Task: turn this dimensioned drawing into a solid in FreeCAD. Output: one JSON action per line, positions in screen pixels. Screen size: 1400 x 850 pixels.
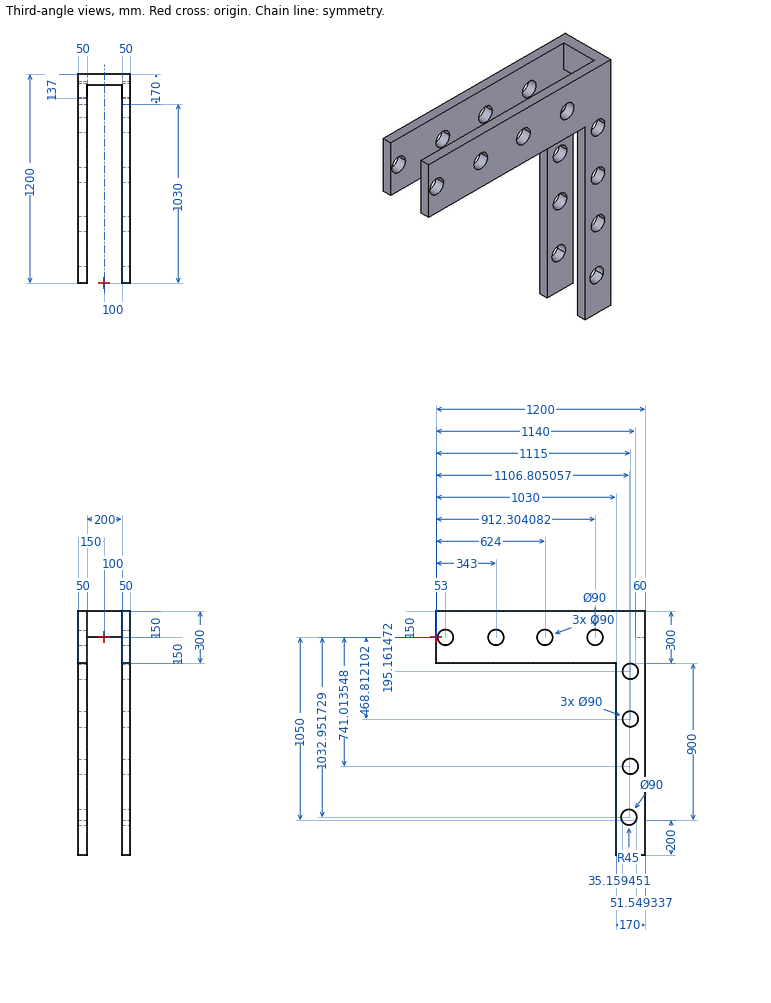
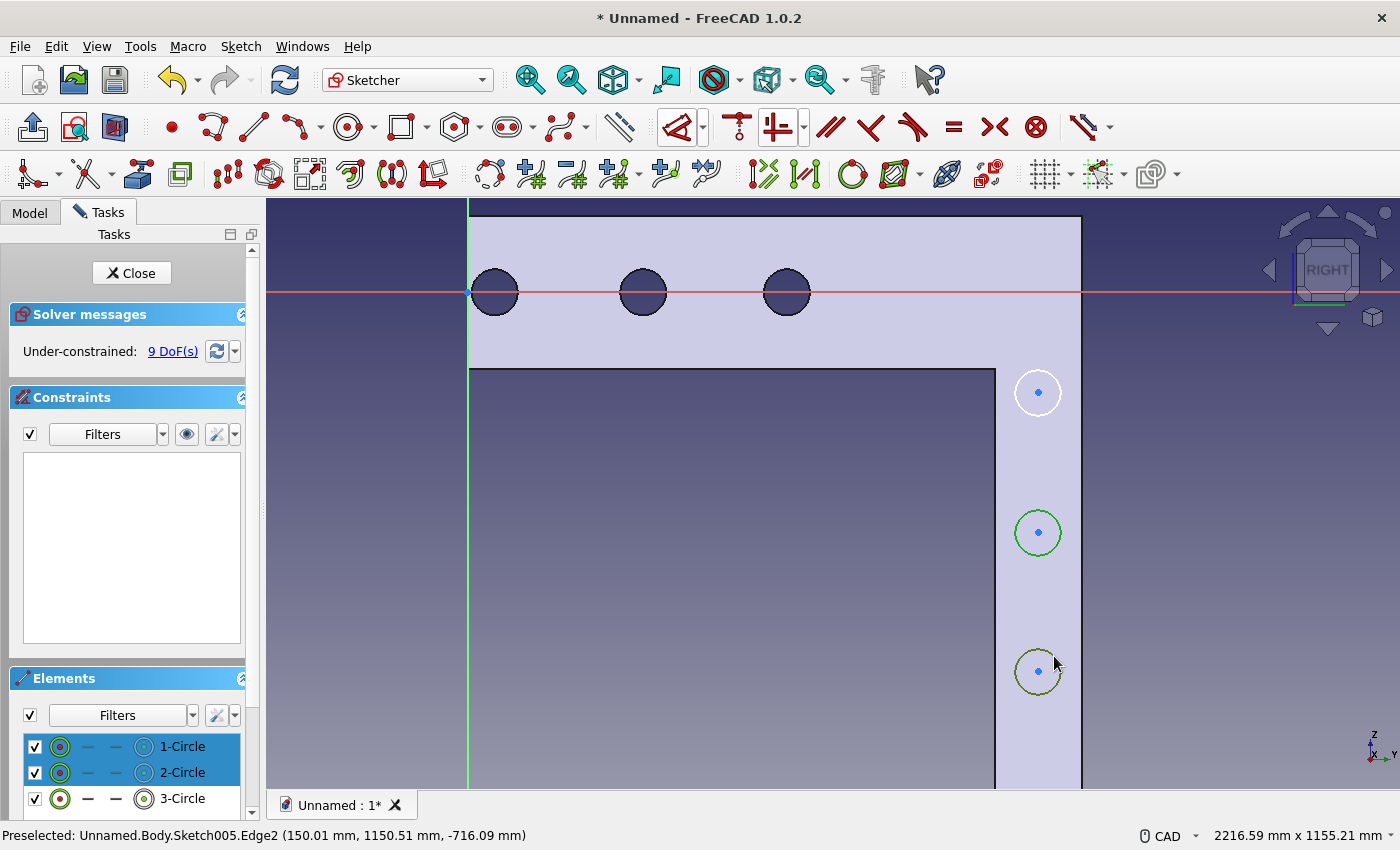
{"action": "left_click", "coordinate": [1054, 377]}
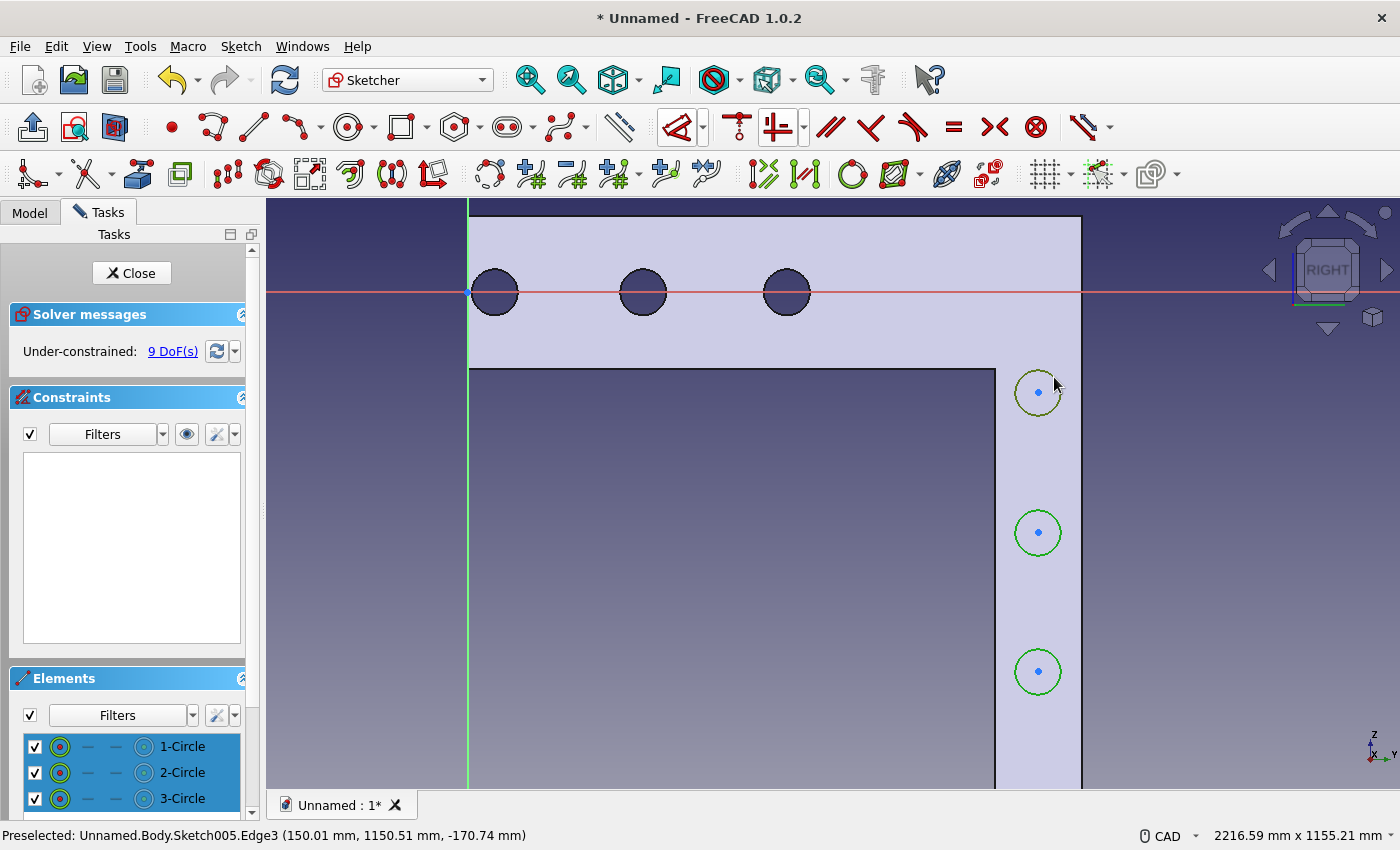
{"action": "left_click", "coordinate": [954, 128]}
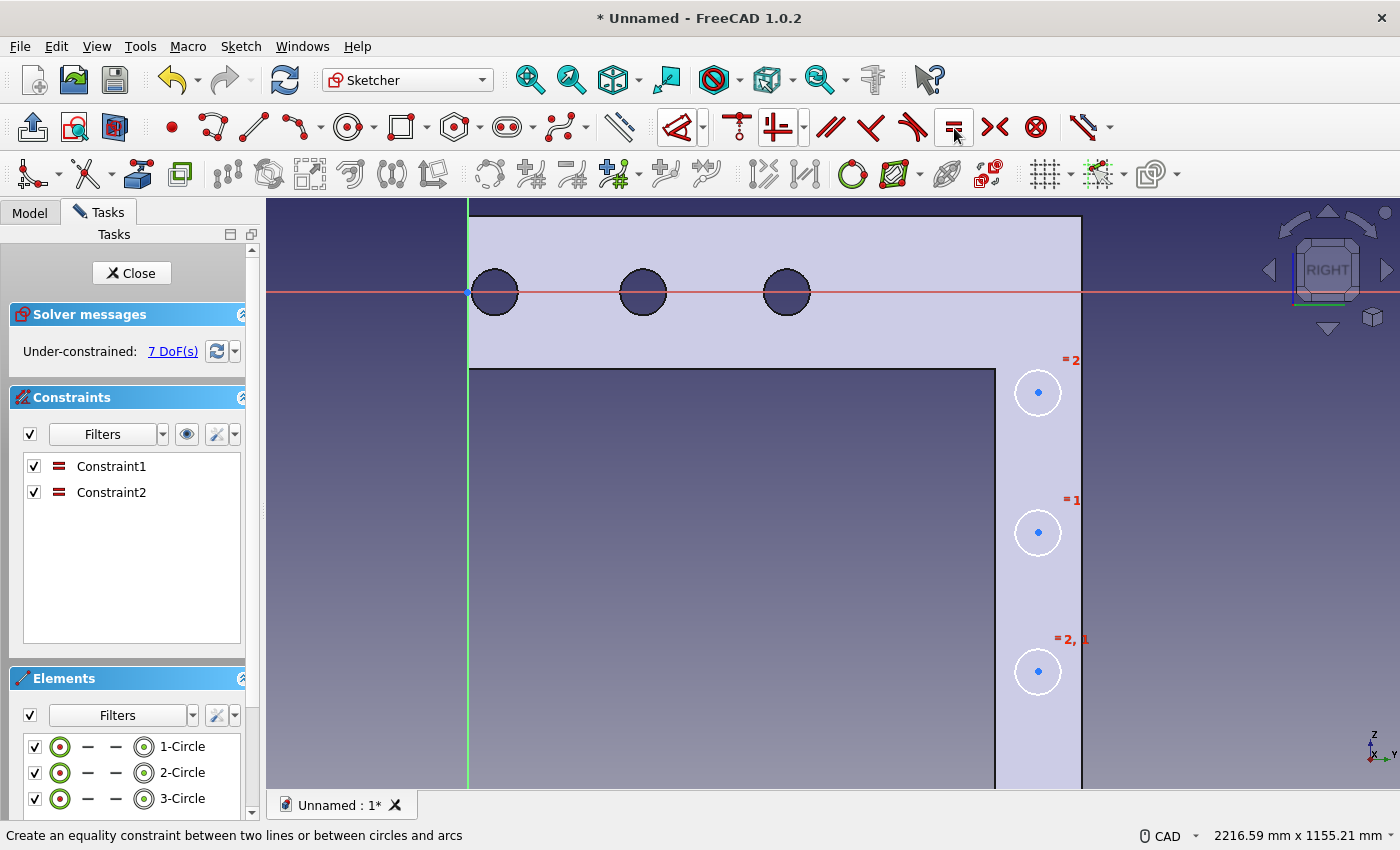
{"action": "left_click", "coordinate": [1038, 533]}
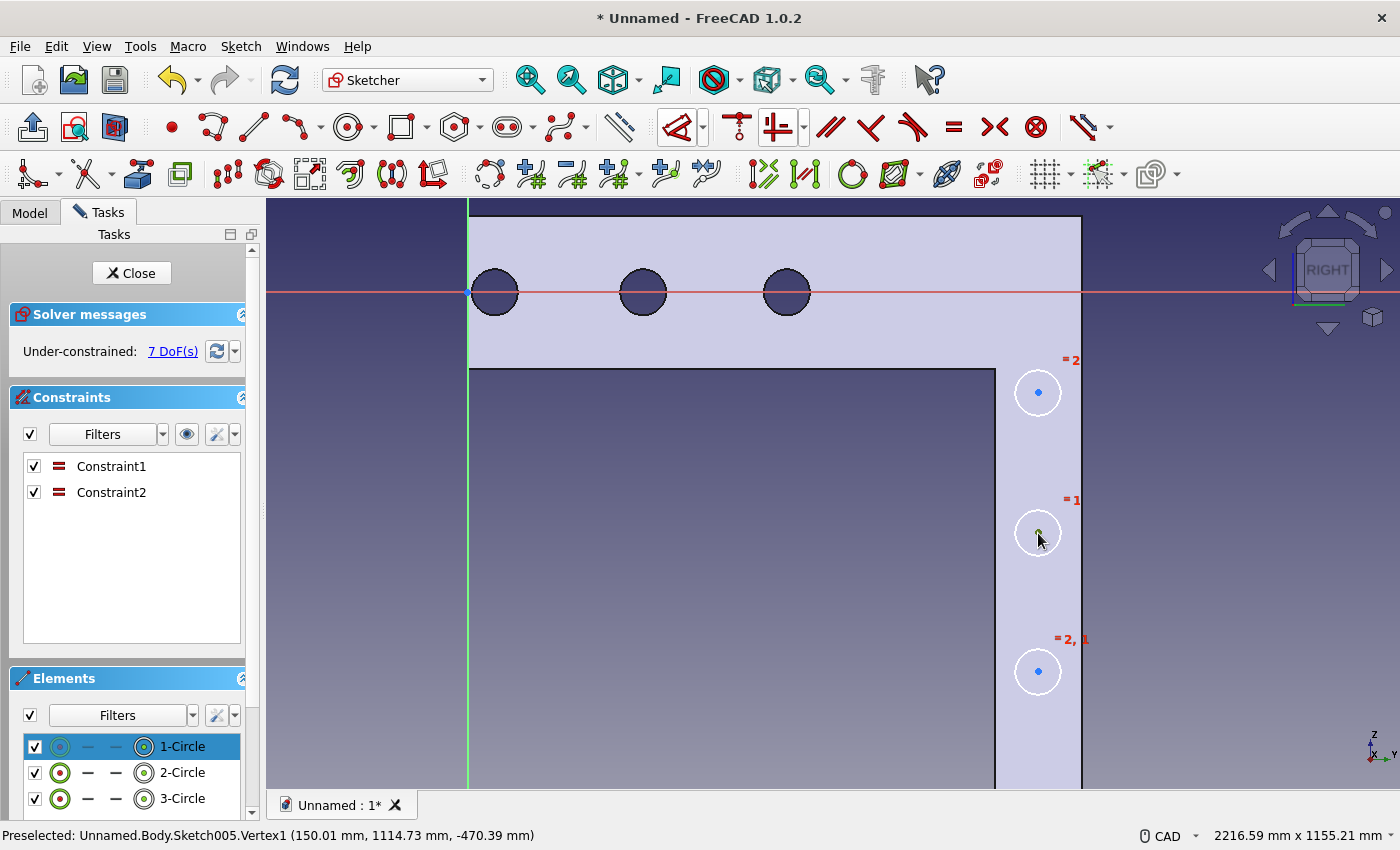
{"action": "left_click", "coordinate": [1038, 672]}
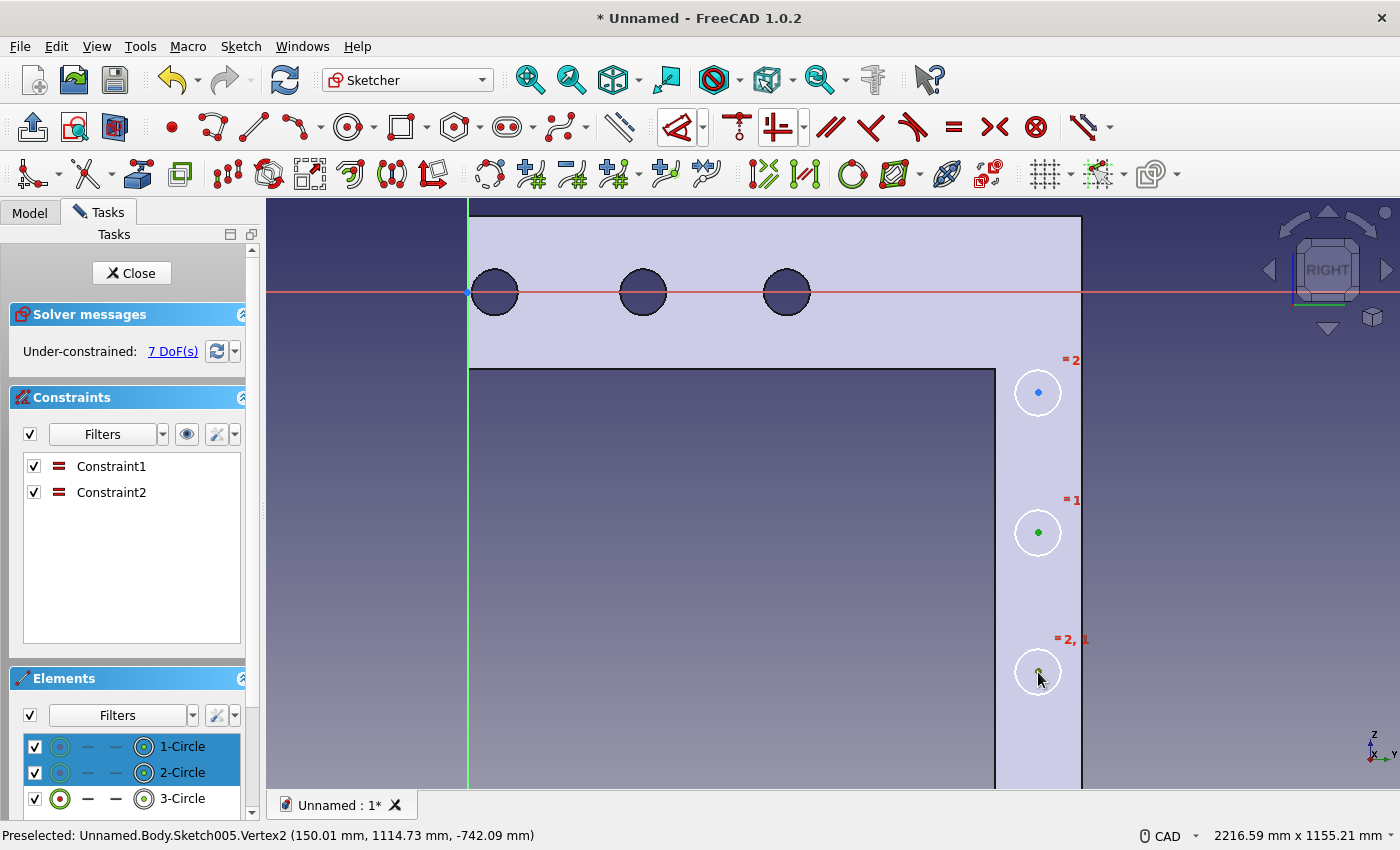
{"action": "left_click", "coordinate": [804, 128]}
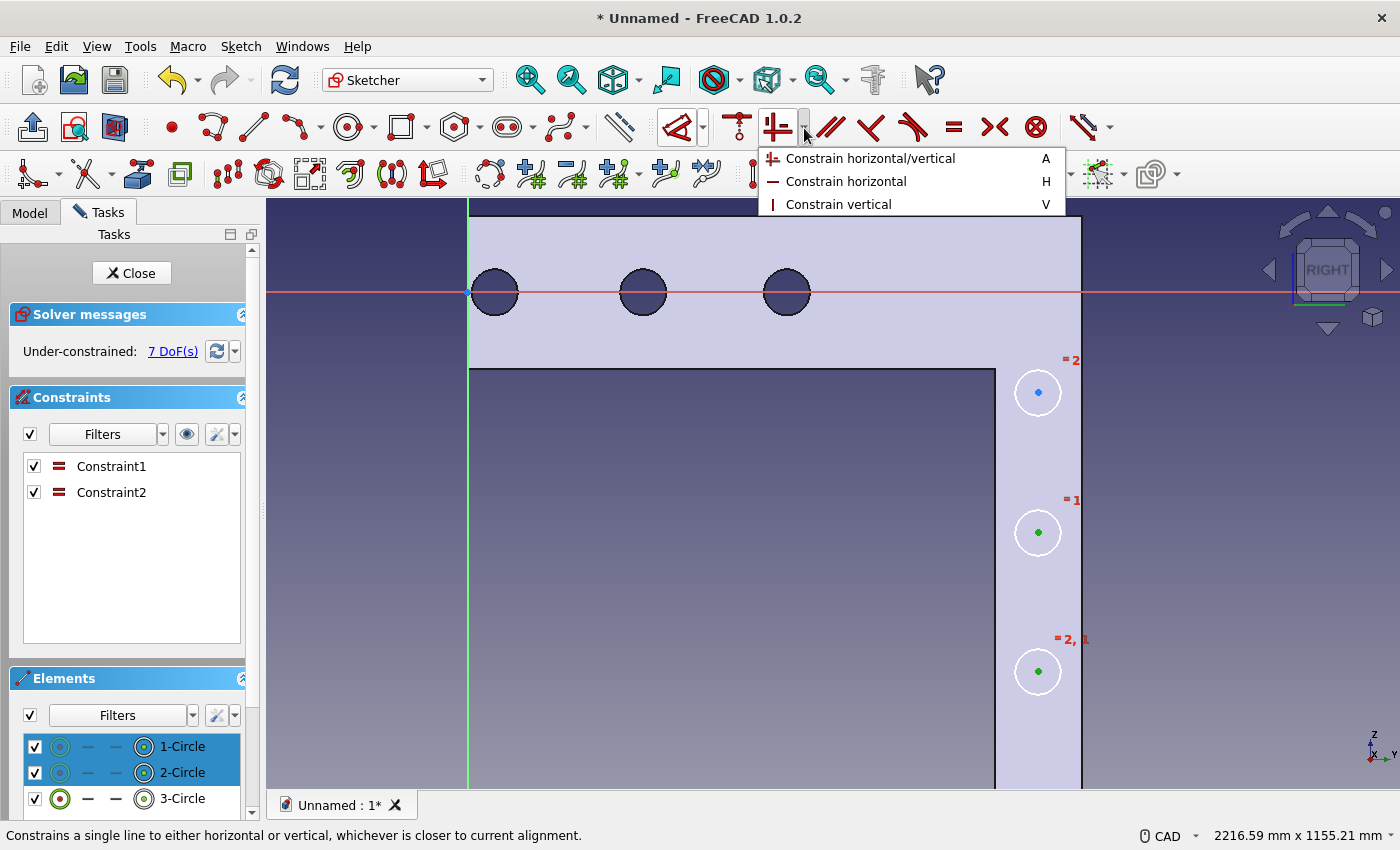
{"action": "left_click", "coordinate": [912, 204]}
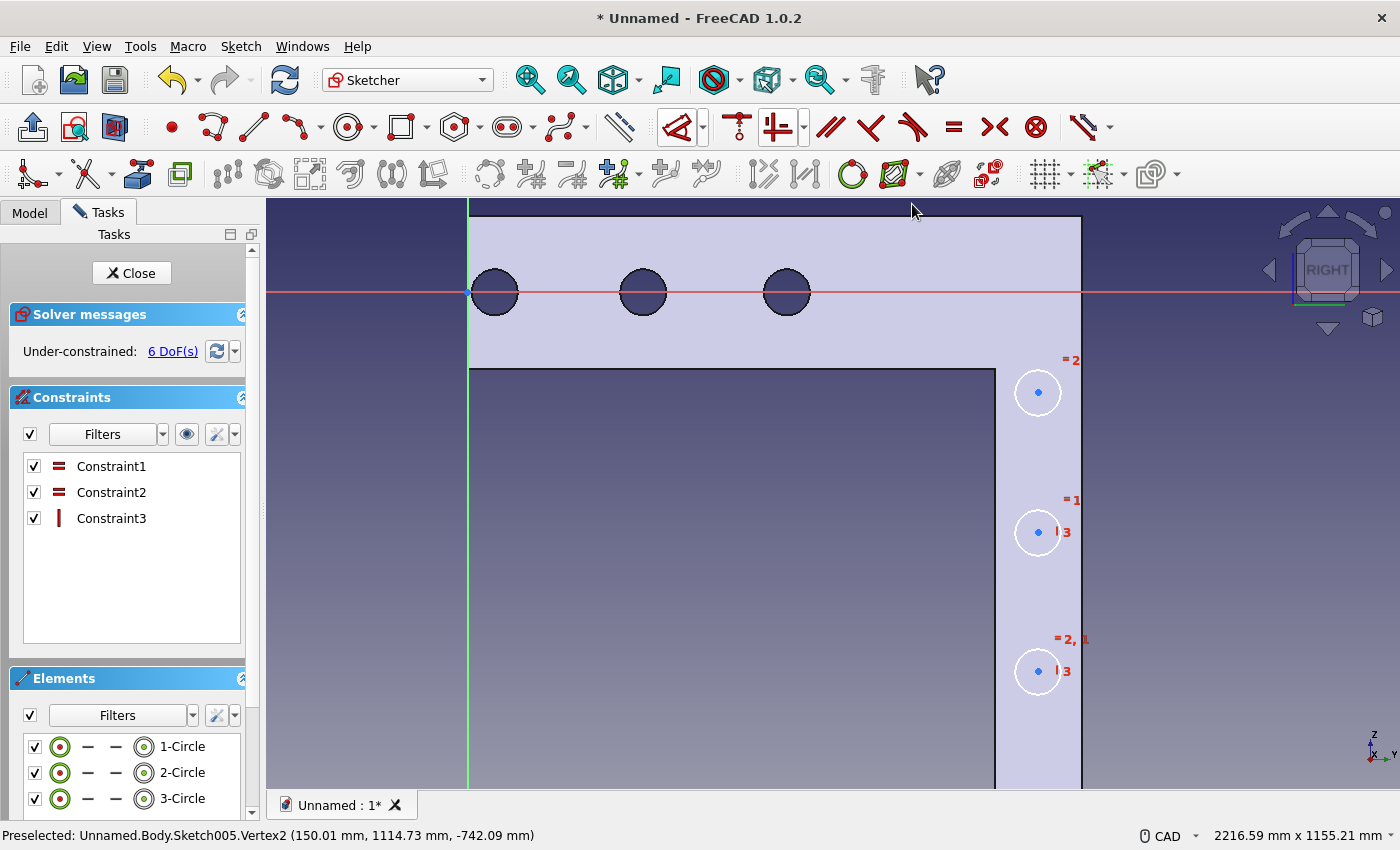
{"action": "left_click", "coordinate": [1038, 533]}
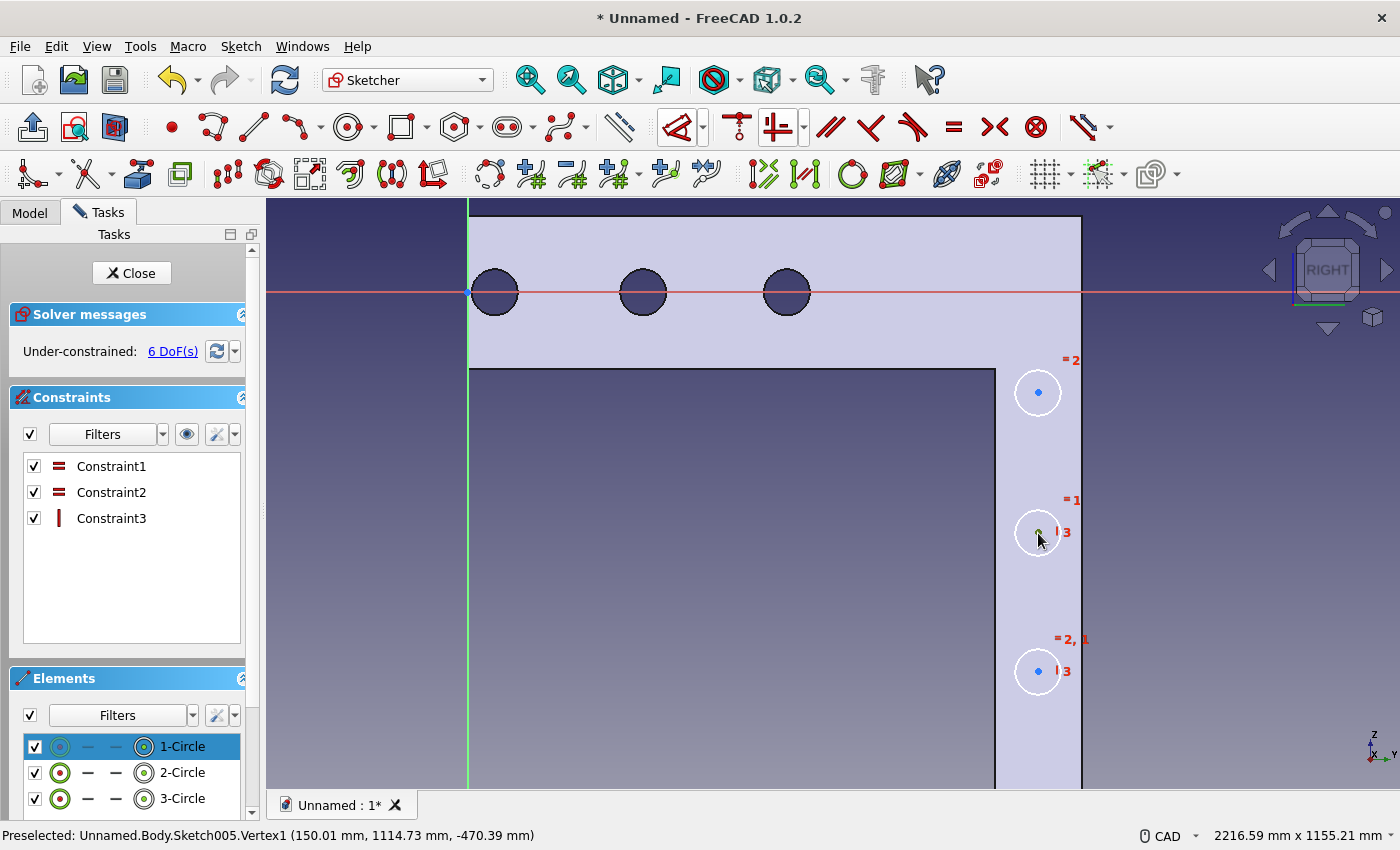
{"action": "left_click", "coordinate": [1038, 393]}